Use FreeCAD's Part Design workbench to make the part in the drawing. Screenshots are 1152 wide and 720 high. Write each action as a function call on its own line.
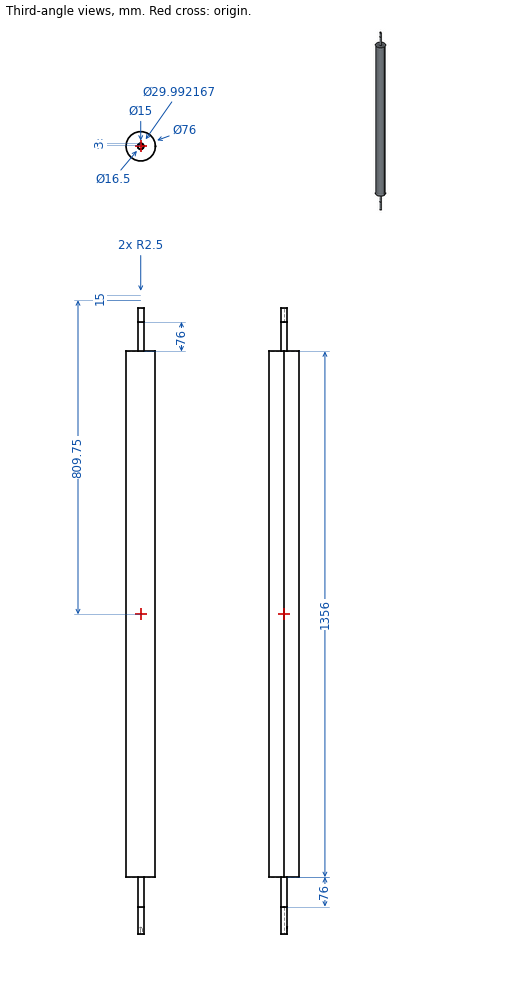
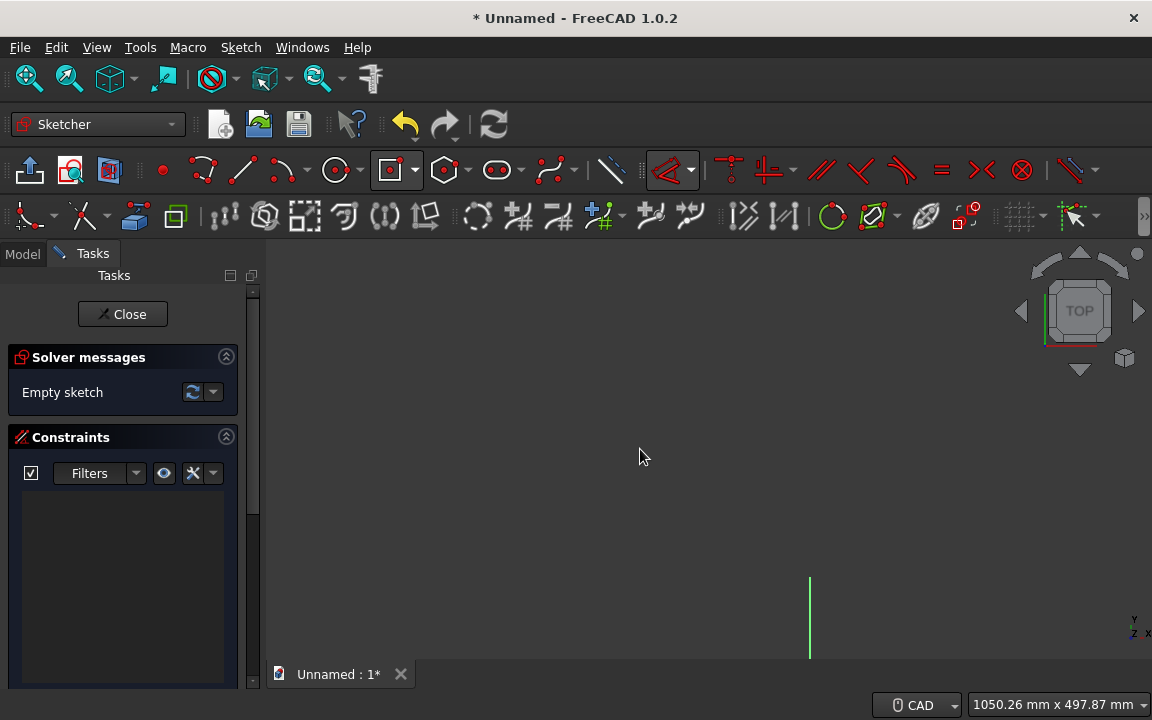
scroll(640, 449, down, 5)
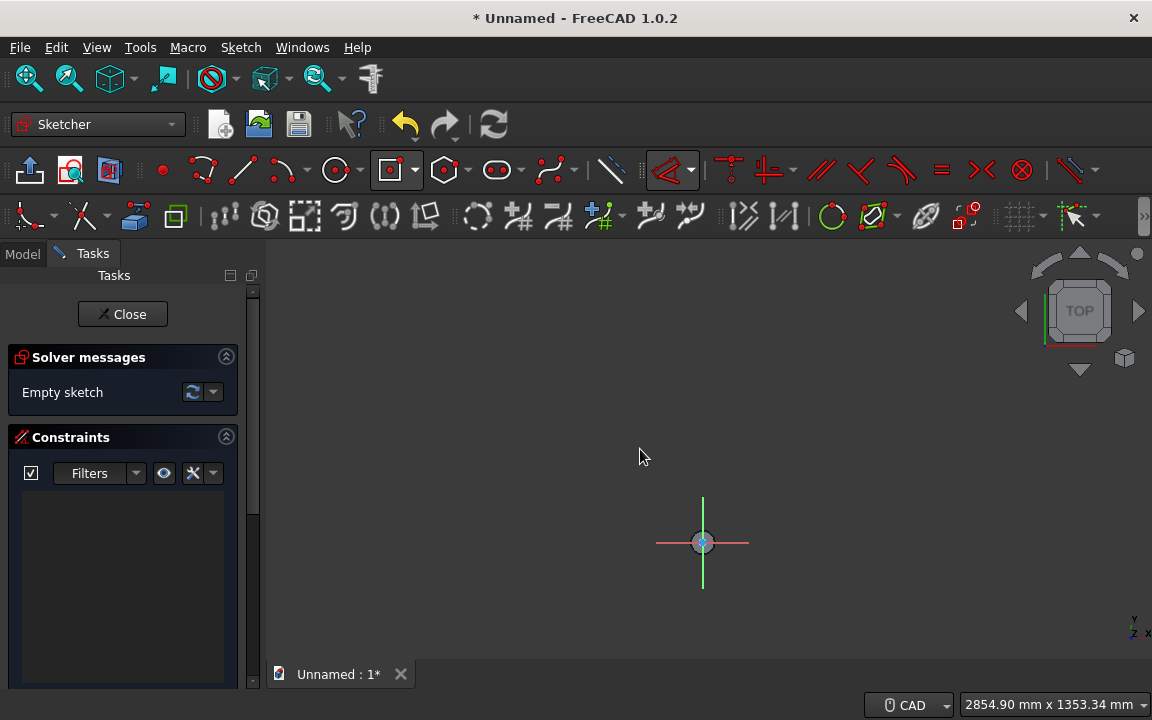
scroll(706, 547, up, 15)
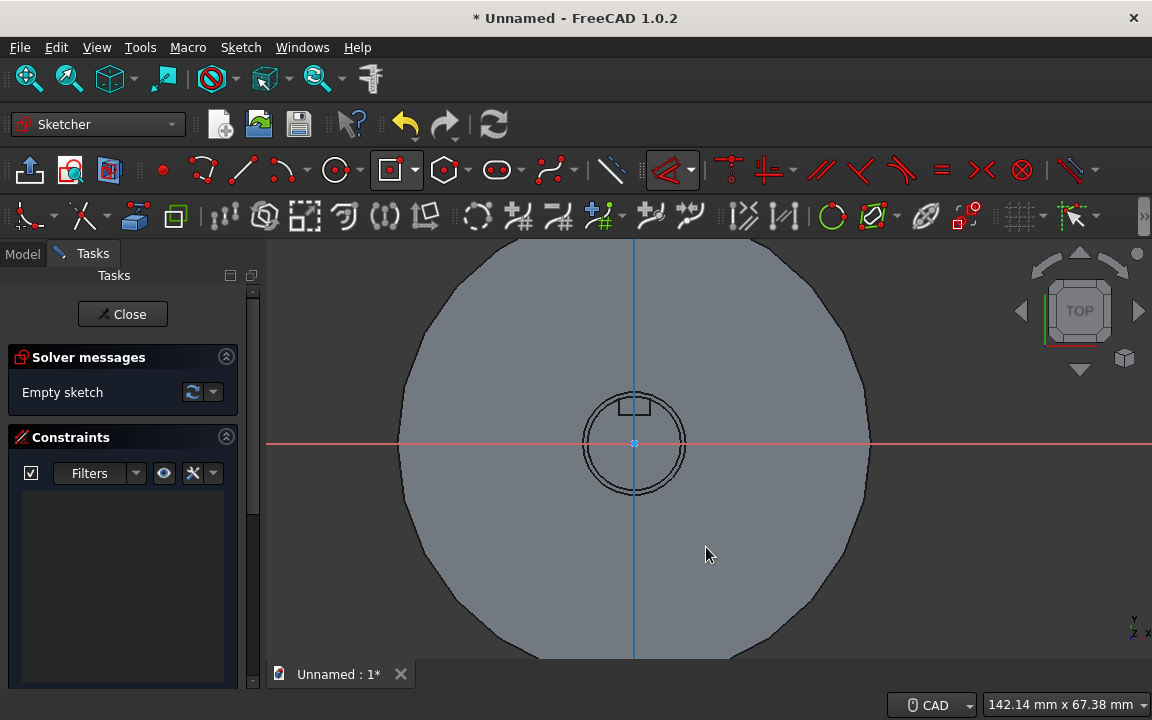
scroll(621, 432, up, 2)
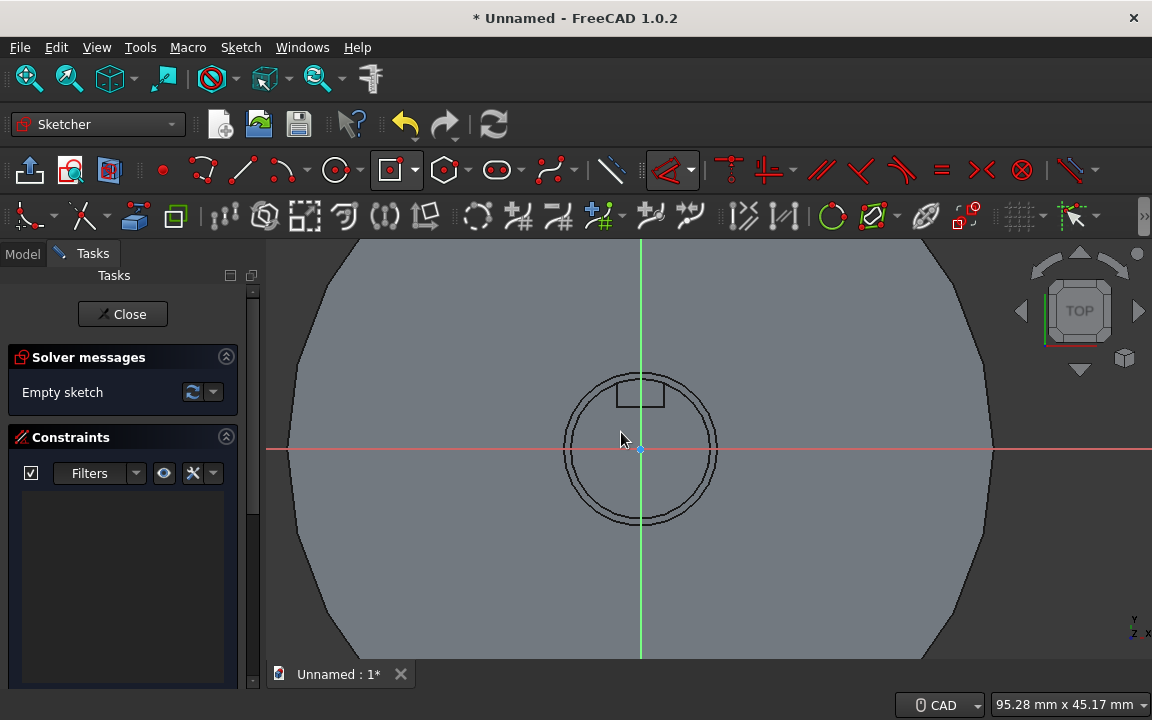
click(336, 170)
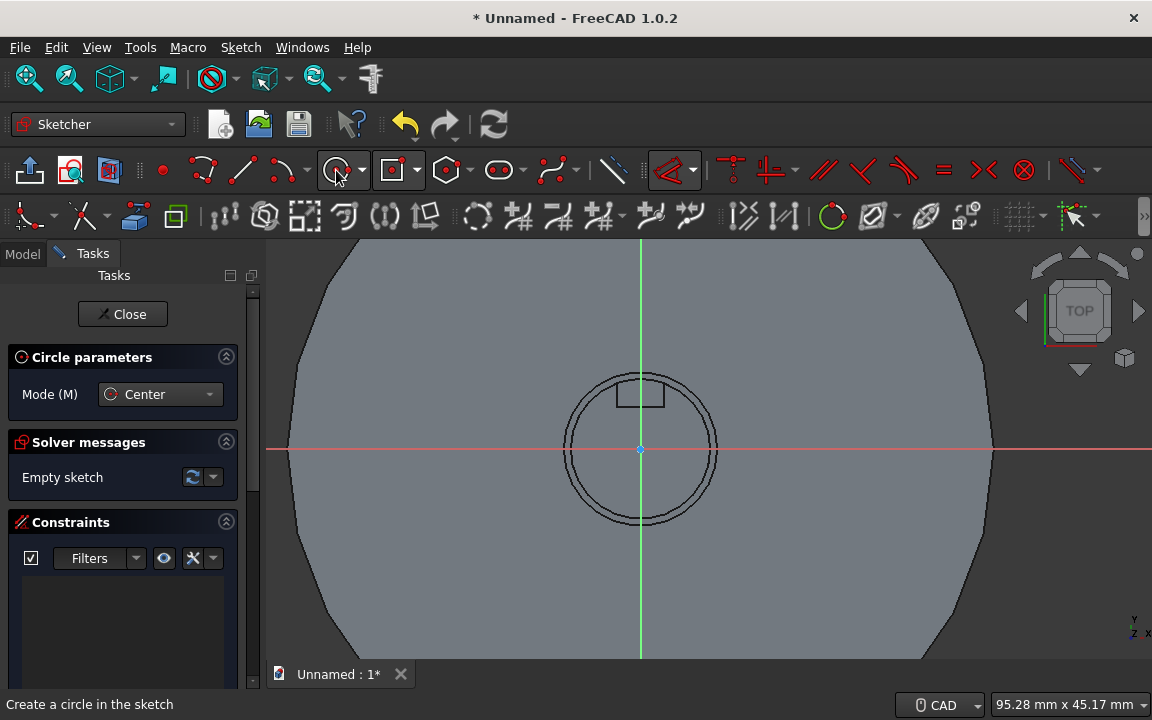
click(641, 449)
click(739, 350)
key(Escape)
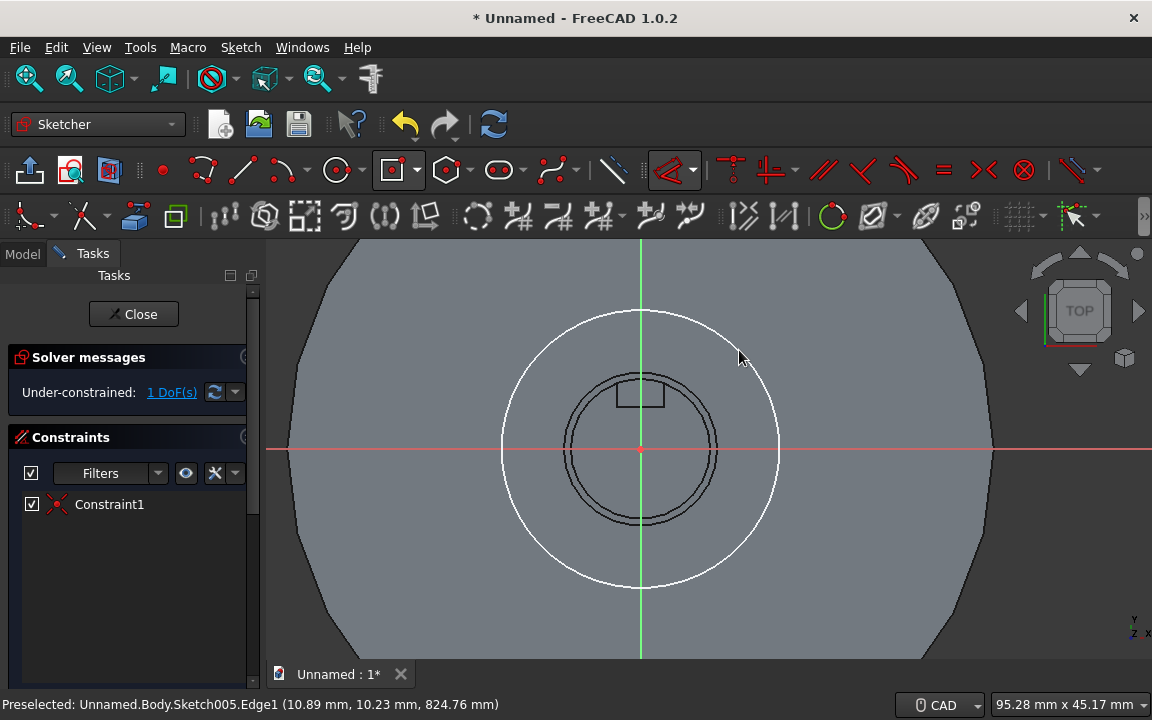
click(738, 350)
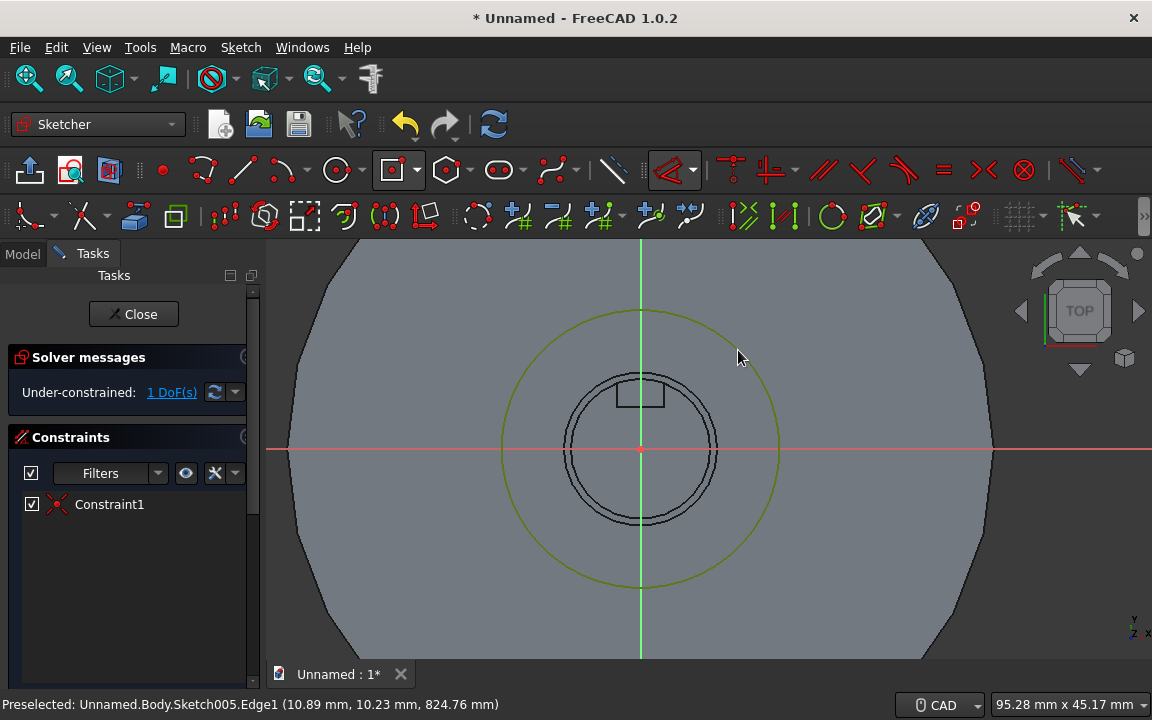
key(k)
key(o)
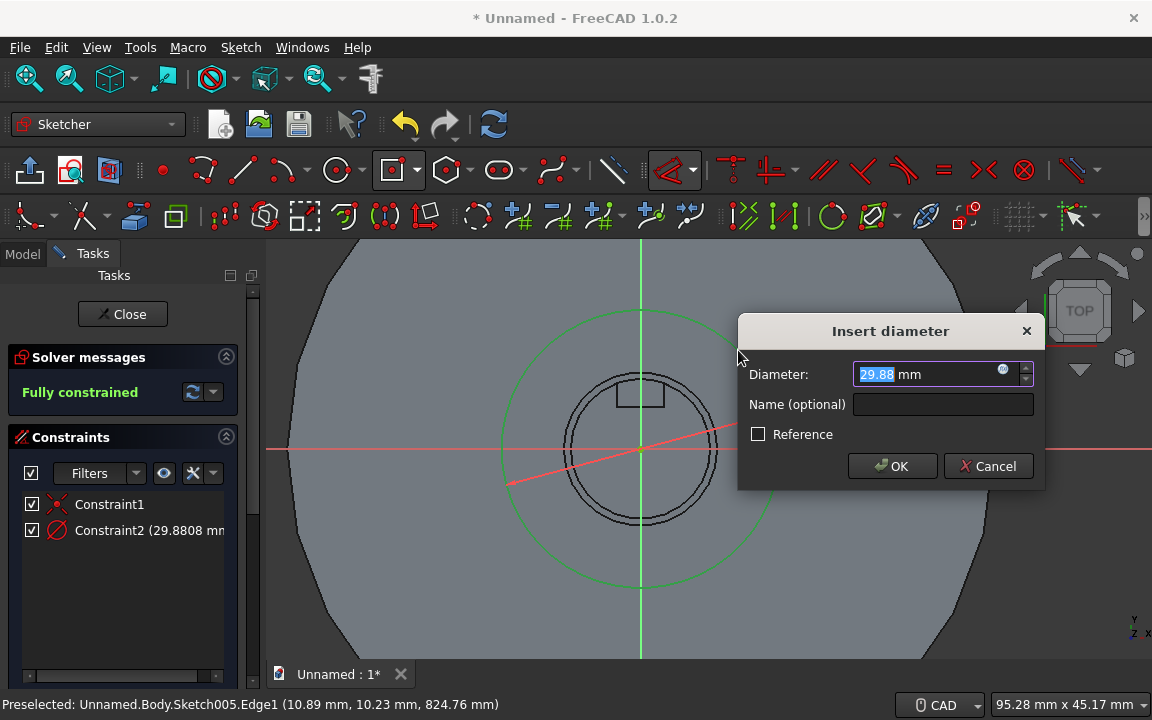
text(29.992167)
key(Return)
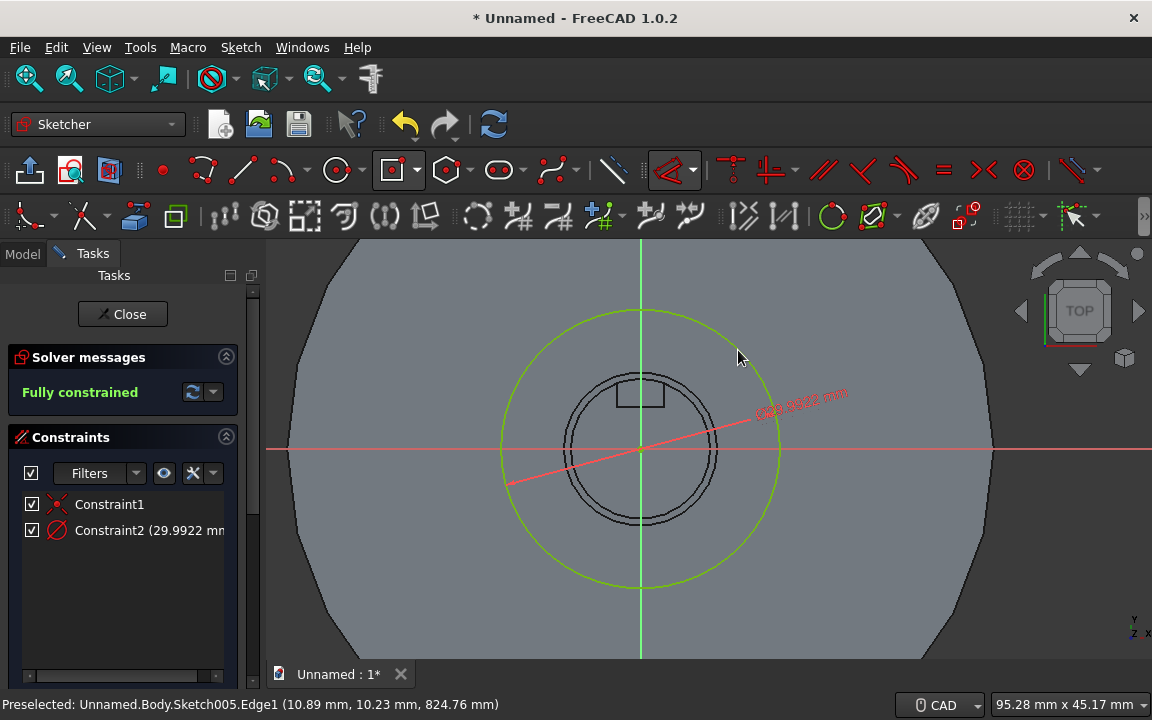
click(123, 314)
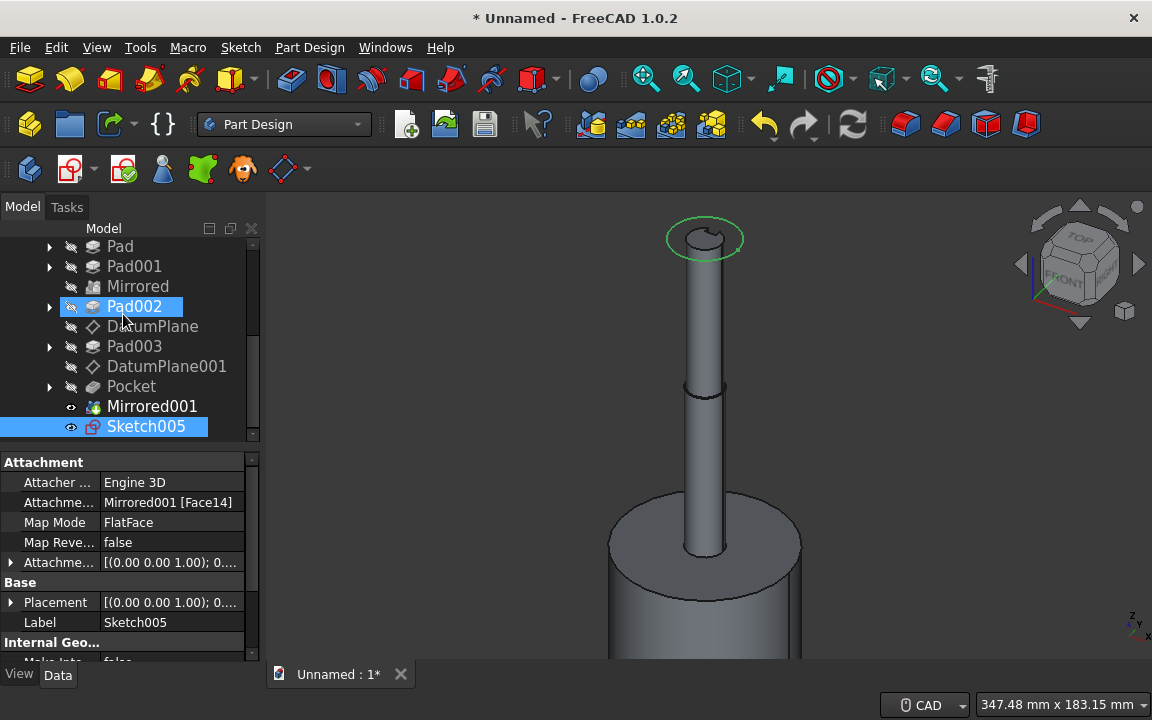
click(292, 80)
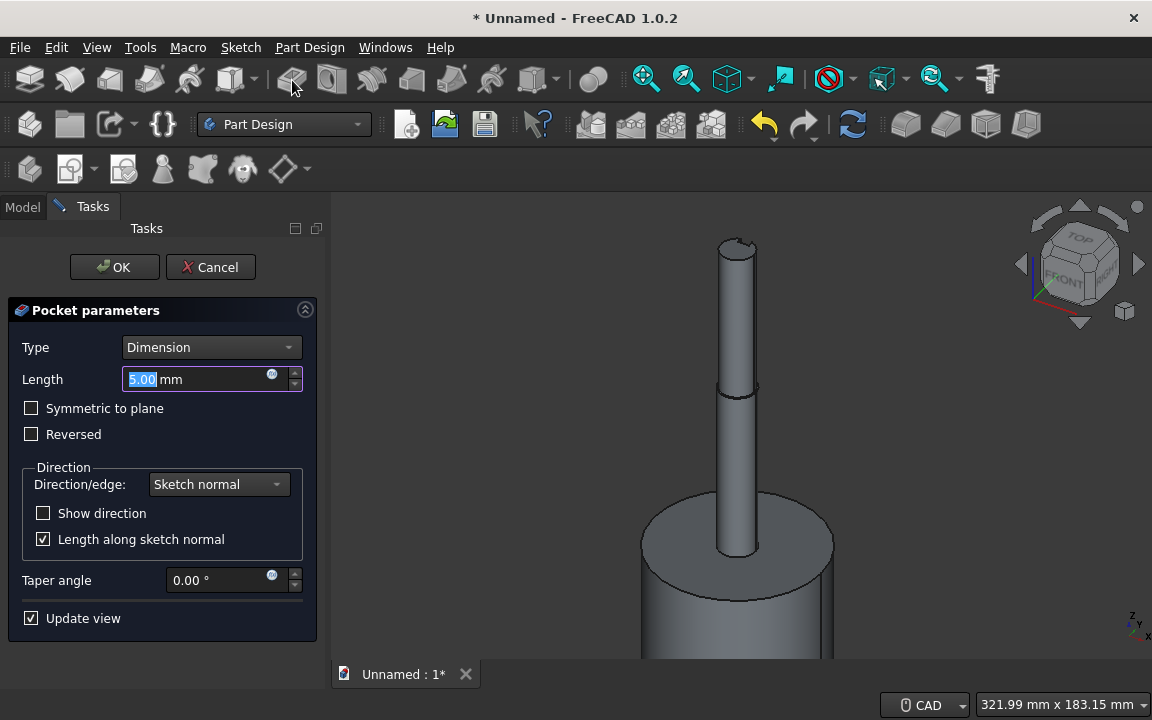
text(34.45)
key(Tab)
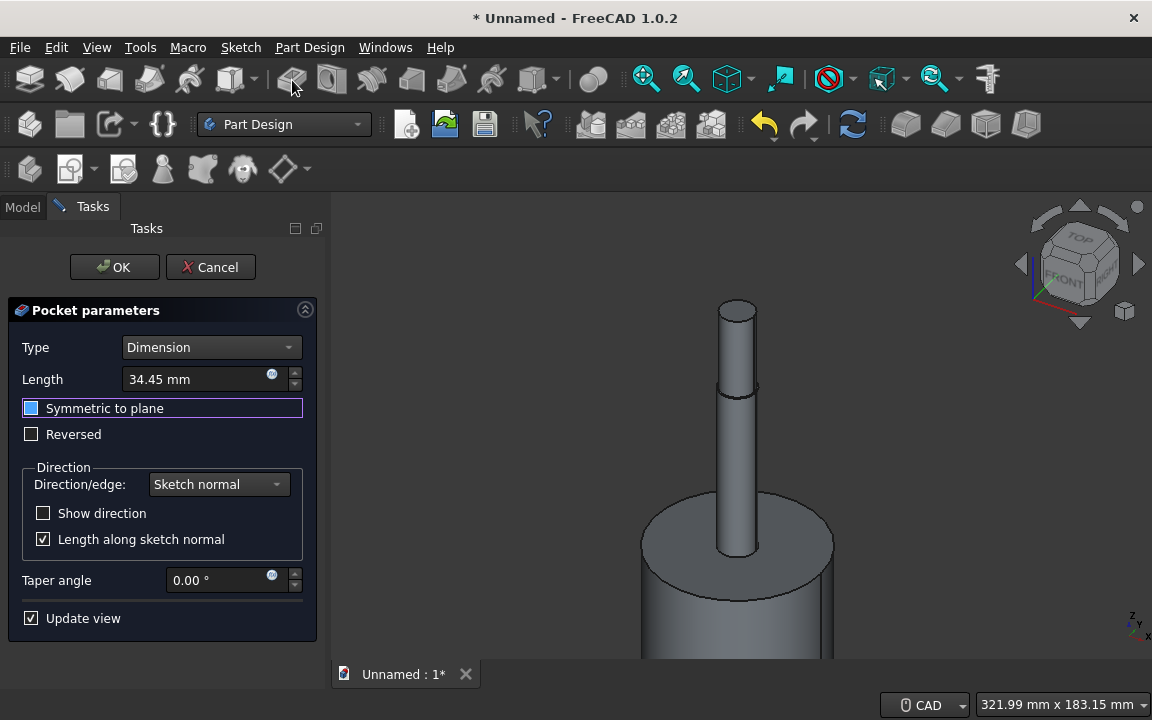
click(115, 267)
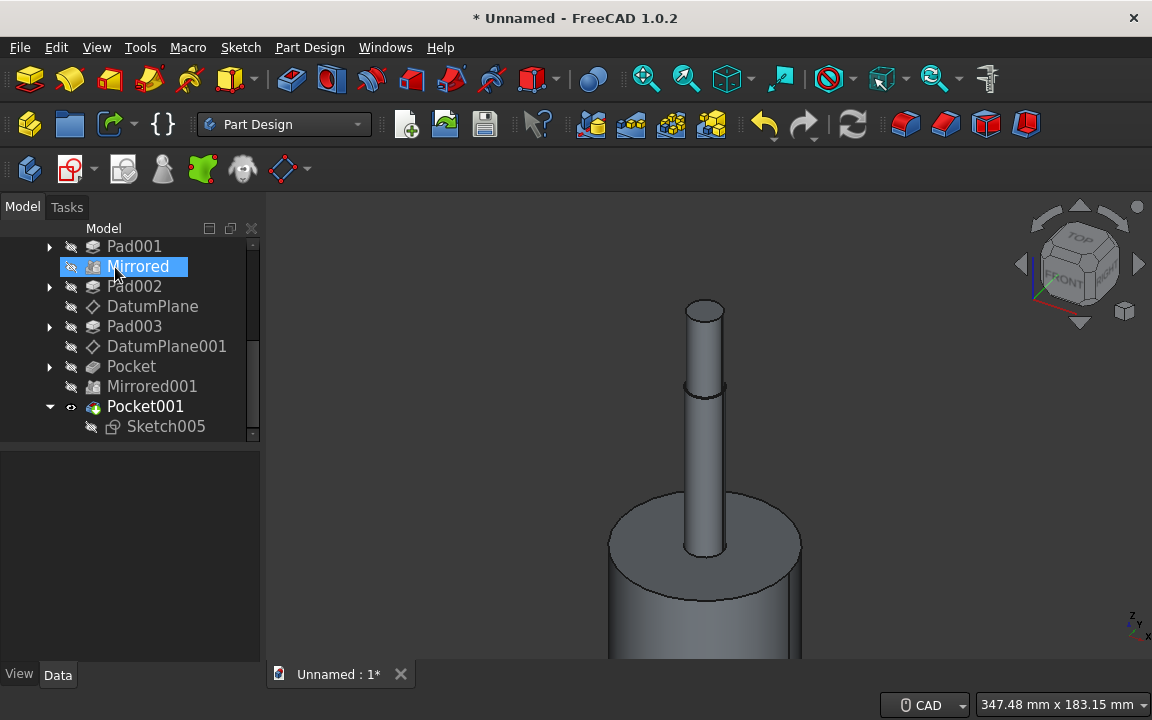
key(0)